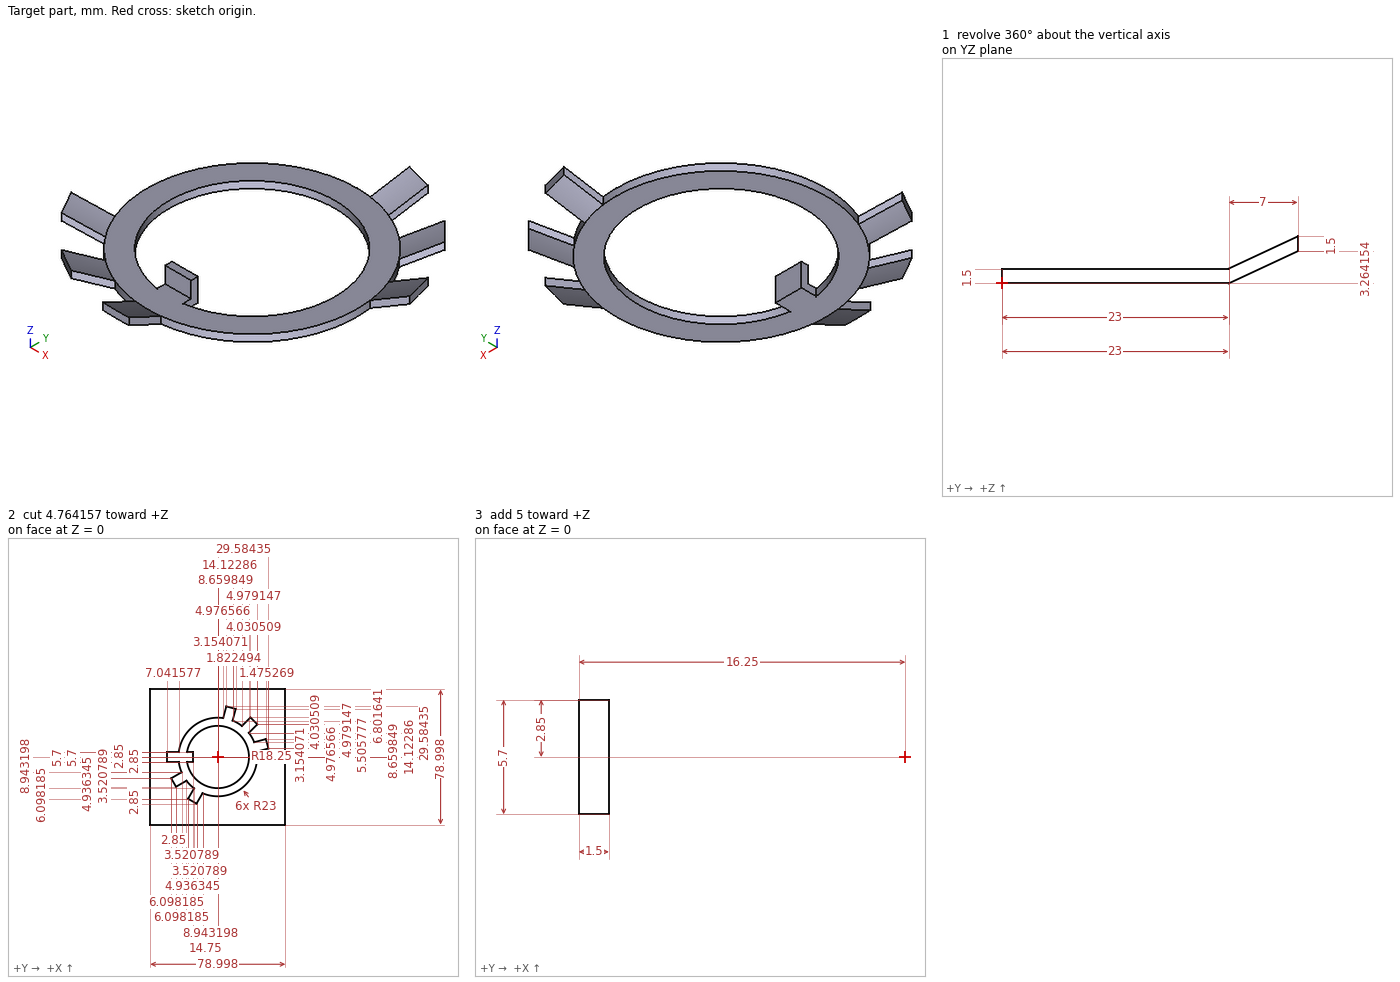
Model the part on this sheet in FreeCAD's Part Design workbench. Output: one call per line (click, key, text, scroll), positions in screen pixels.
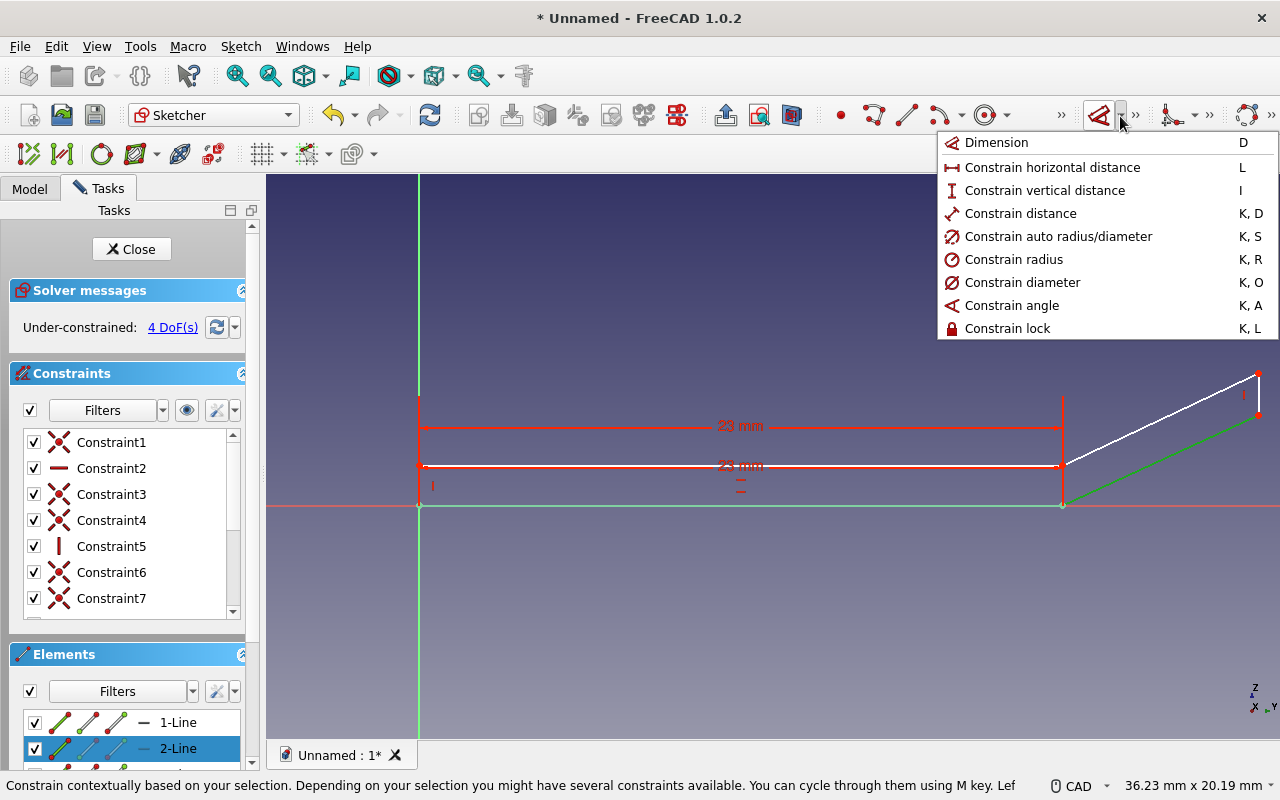
click(1108, 168)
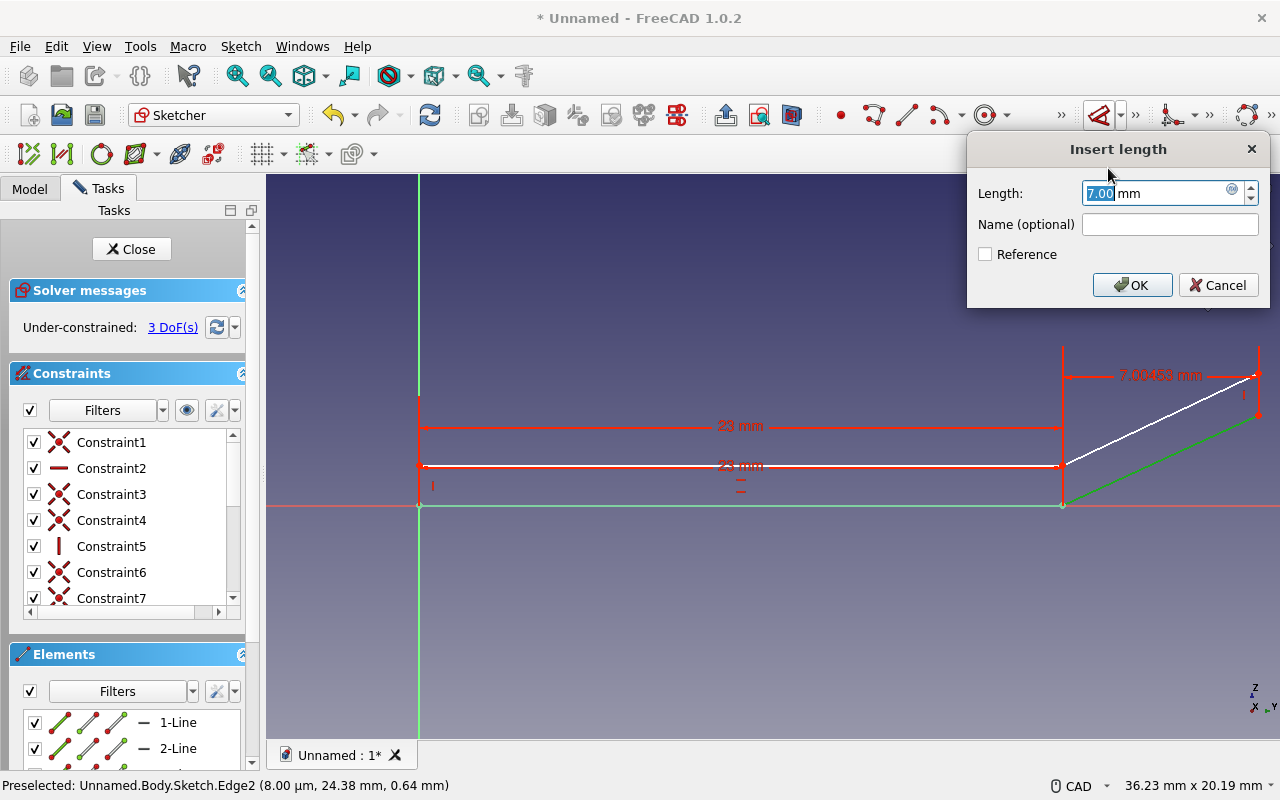
text(7)
key(Return)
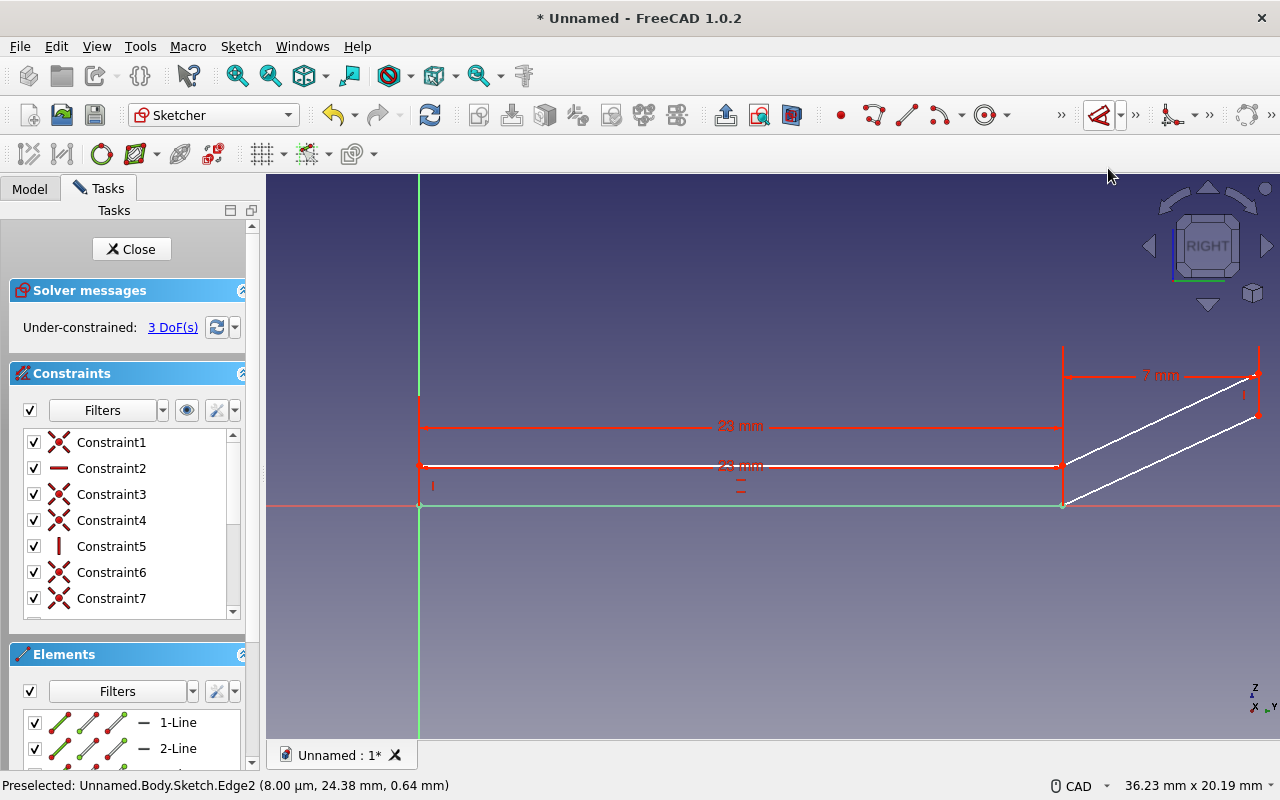
scroll(431, 492, down, 2)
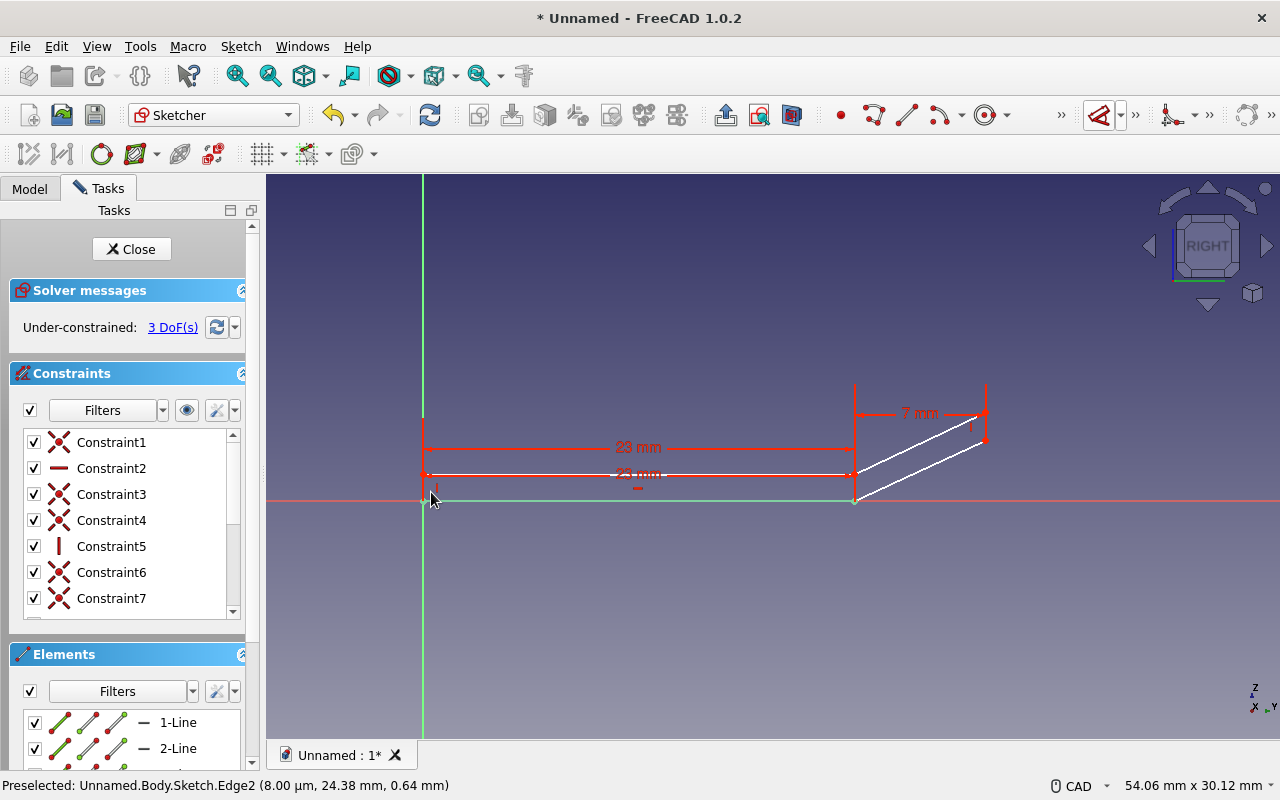
scroll(986, 432, up, 3)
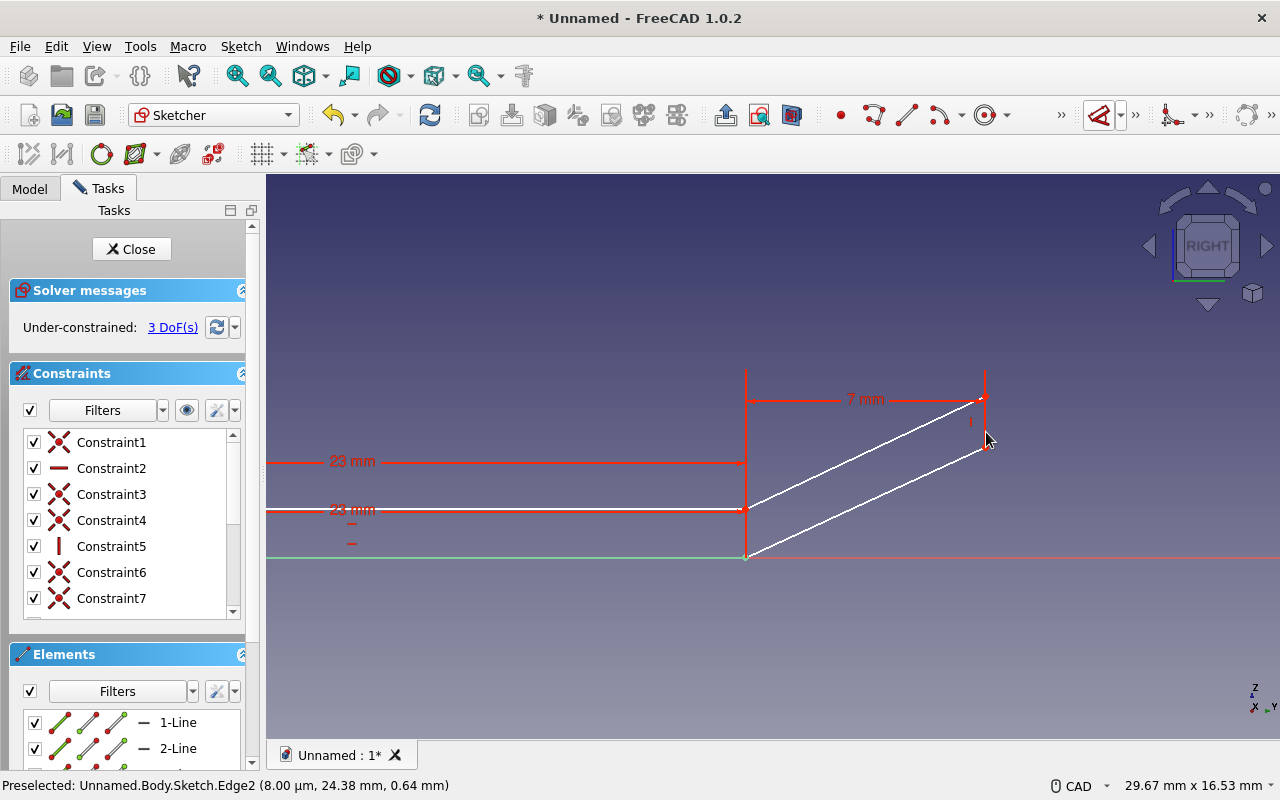
click(985, 432)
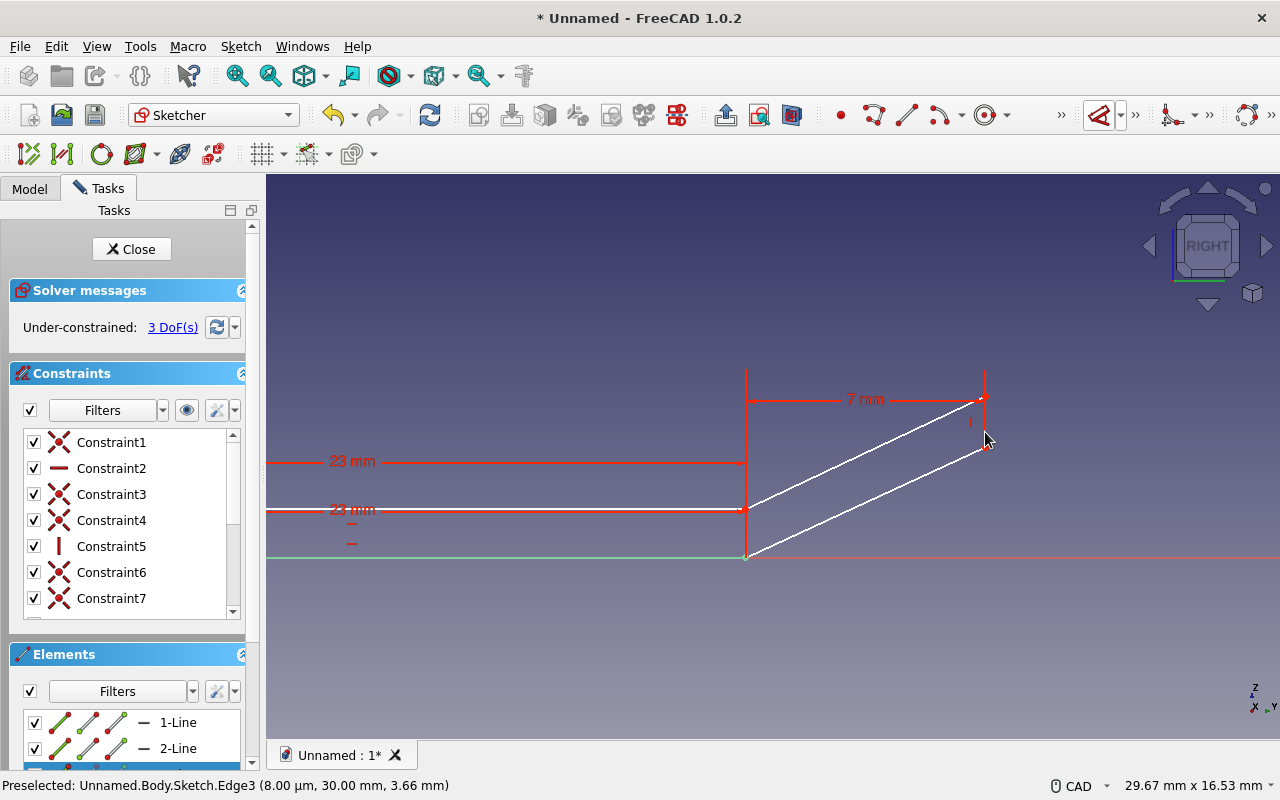
click(1120, 116)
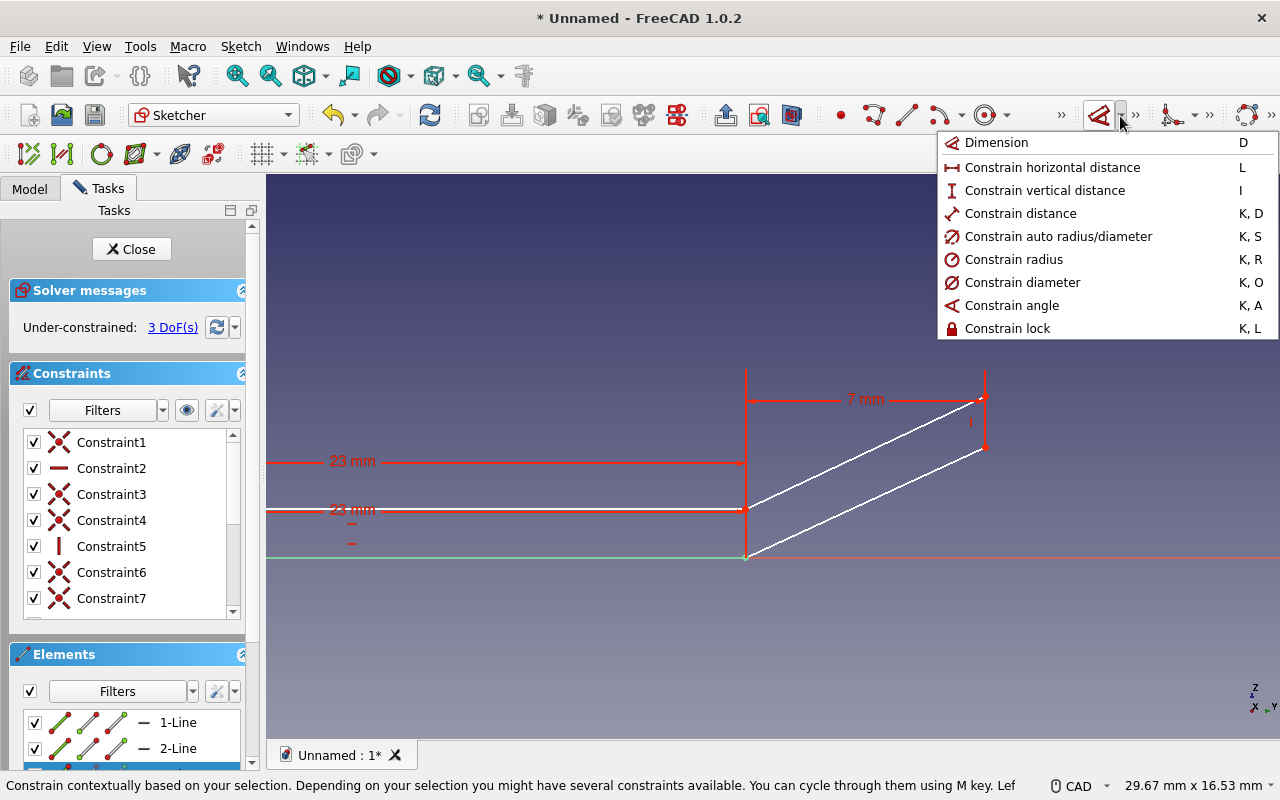
click(1108, 190)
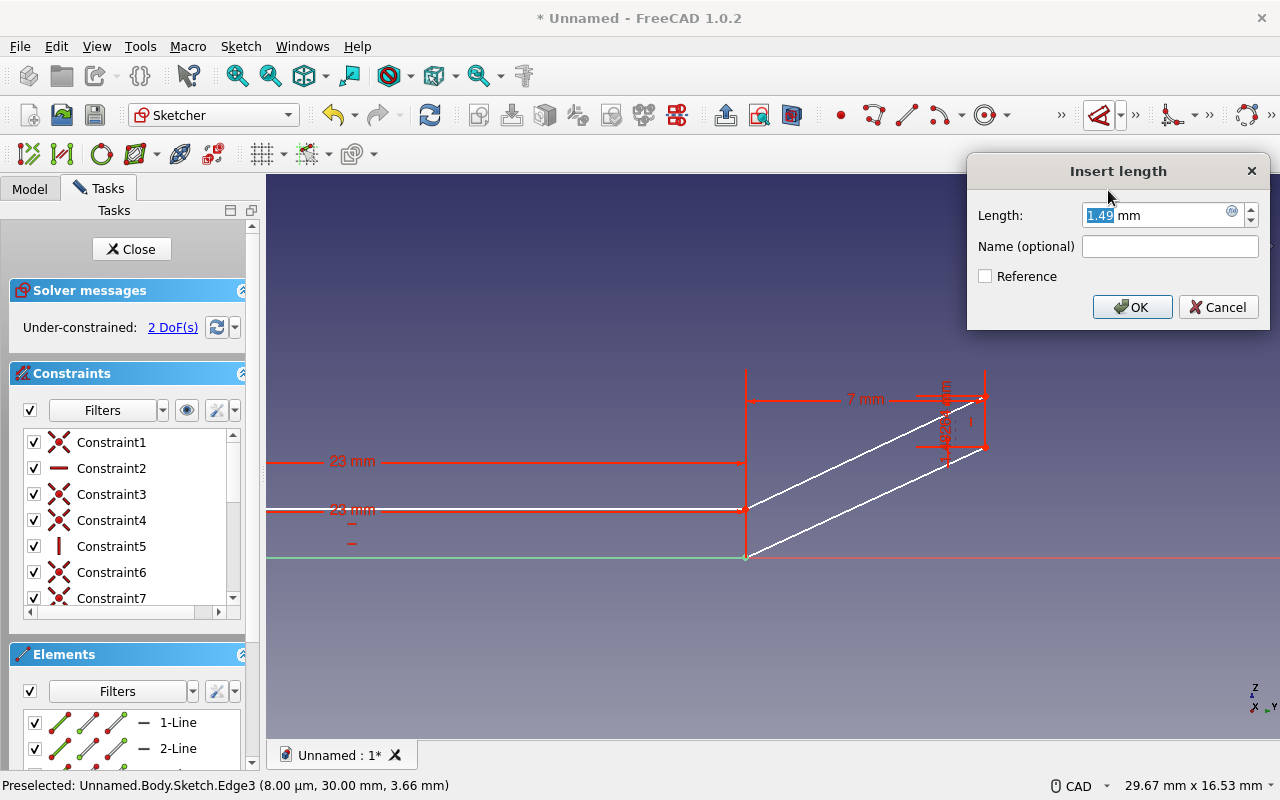
text(1.5)
key(Return)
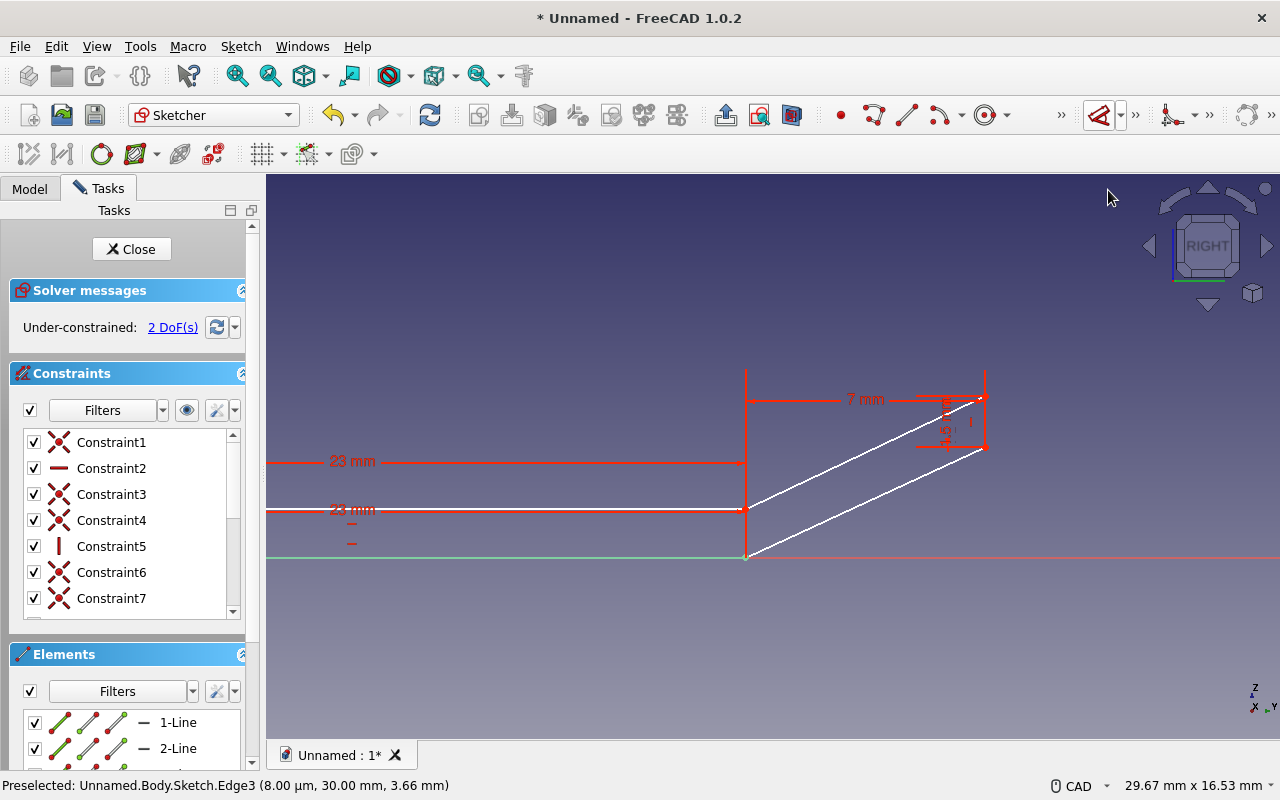
scroll(987, 432, down, 3)